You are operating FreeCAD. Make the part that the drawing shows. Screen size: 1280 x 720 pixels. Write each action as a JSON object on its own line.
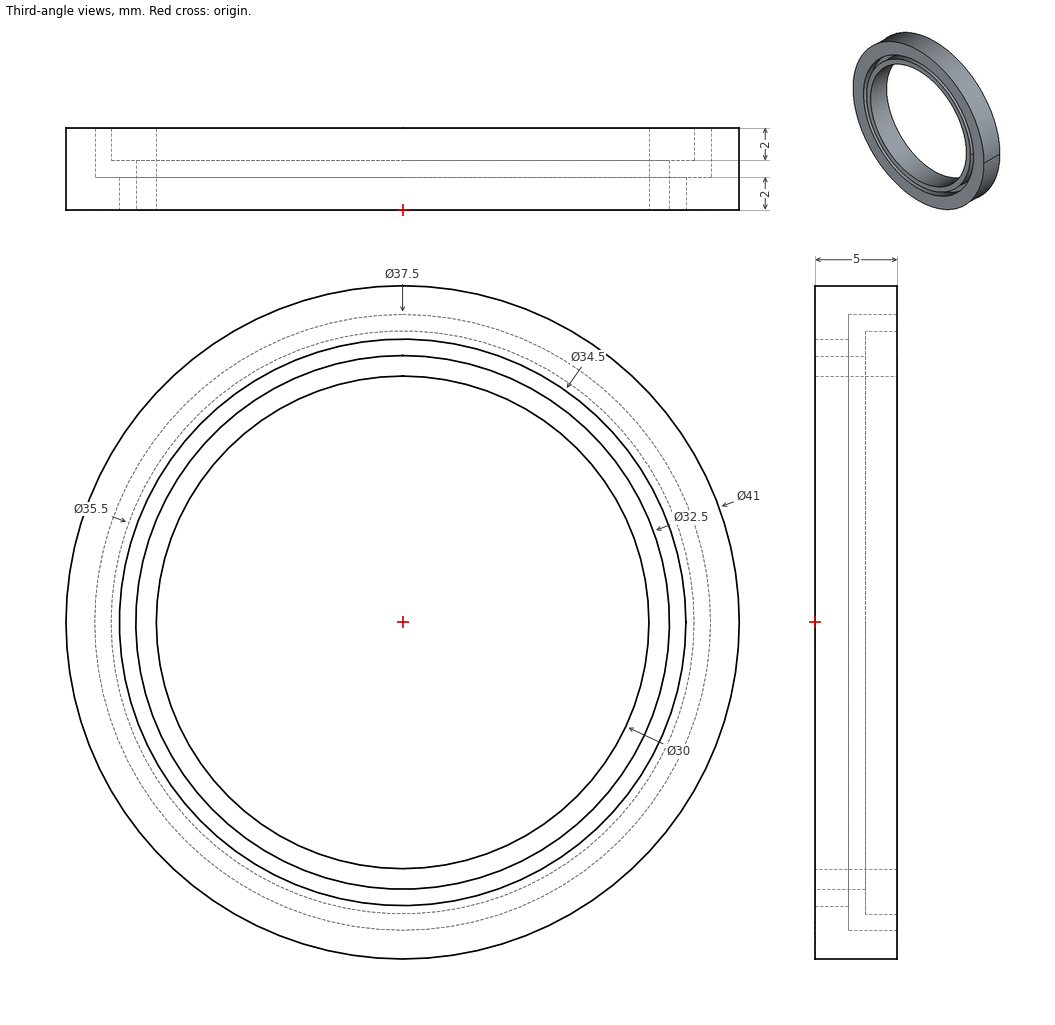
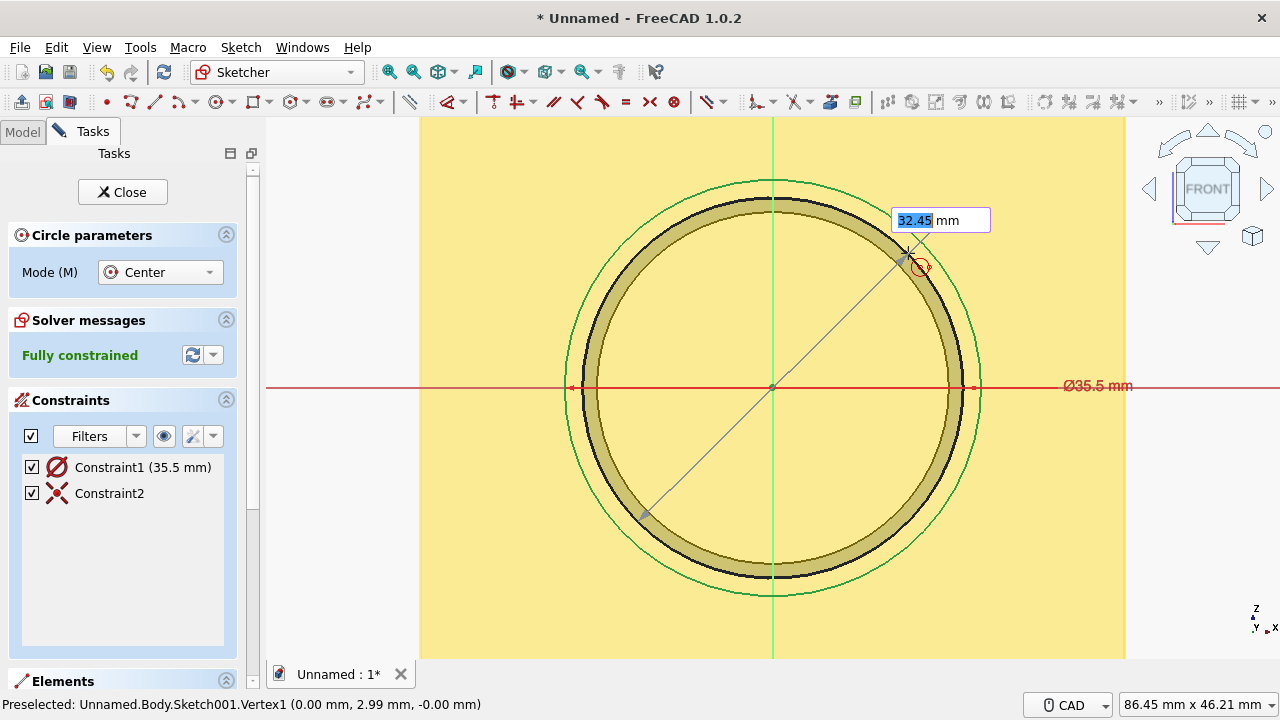
{"action": "type", "text": "32.5"}
{"action": "key", "text": "Return"}
{"action": "key", "text": "Escape"}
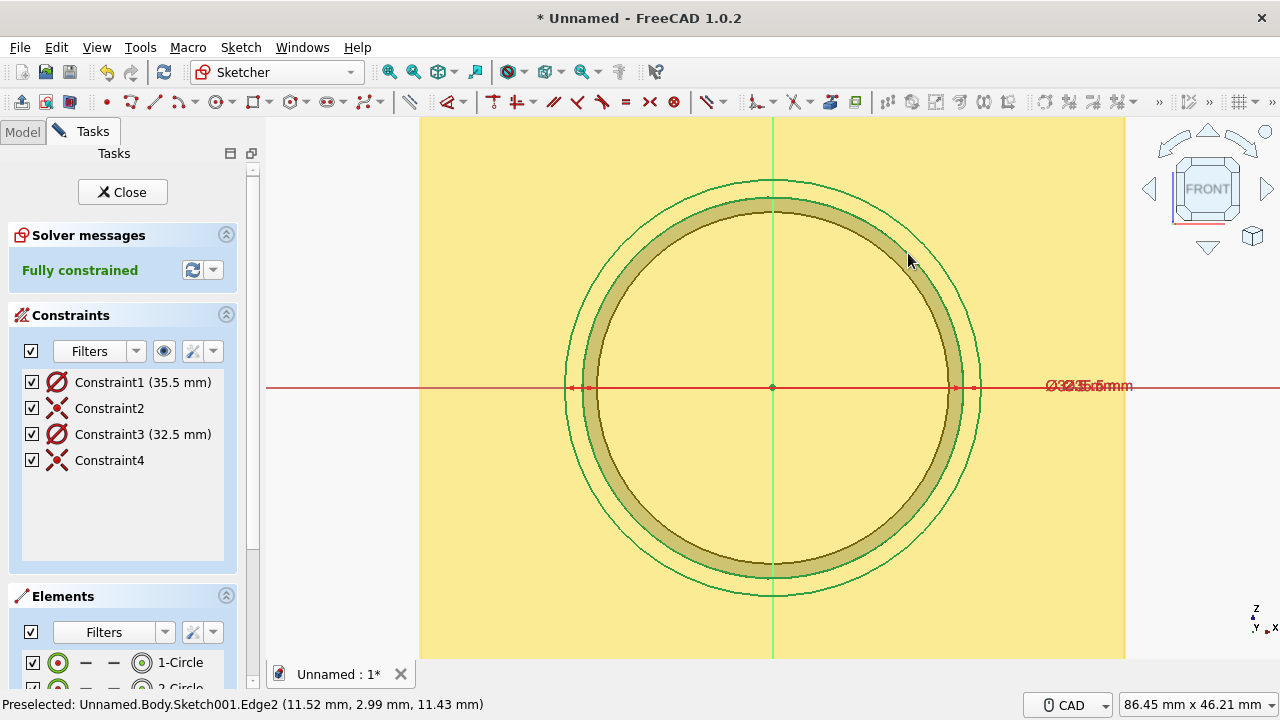
{"action": "left_click", "coordinate": [123, 192]}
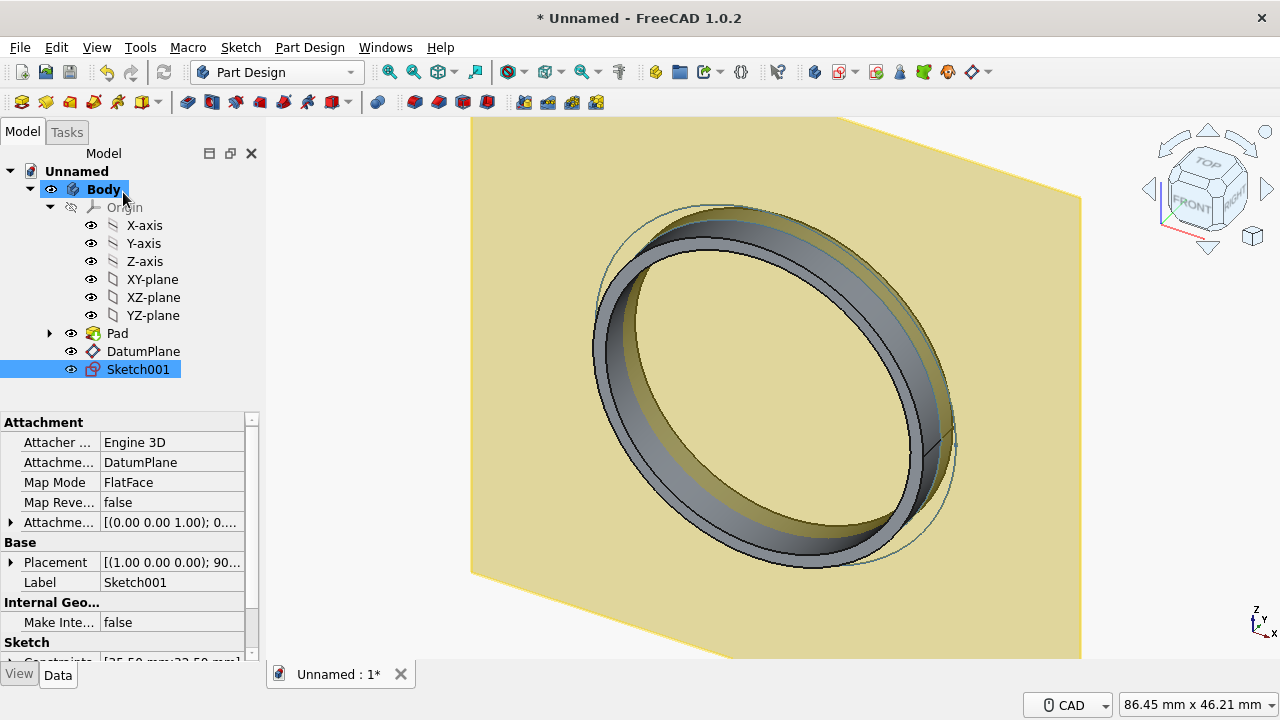
{"action": "left_click", "coordinate": [22, 102]}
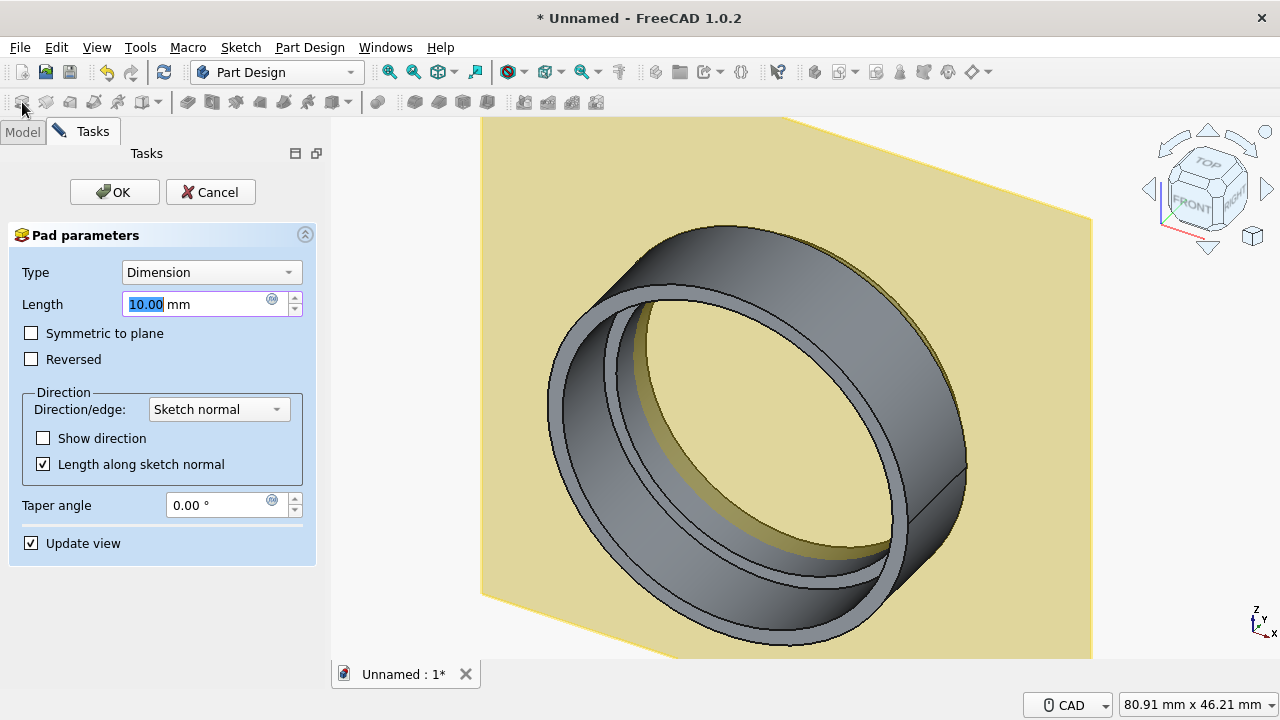
{"action": "type", "text": "2"}
{"action": "key", "text": "Tab"}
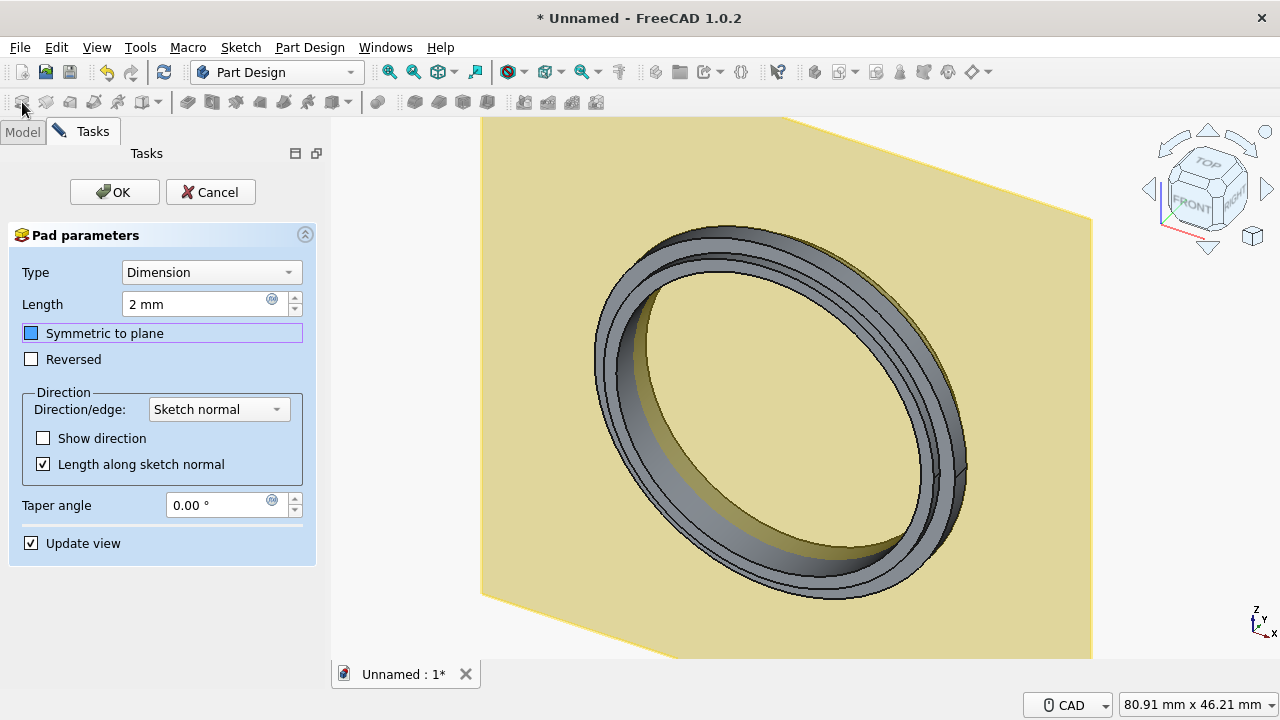
{"action": "left_click", "coordinate": [30, 359]}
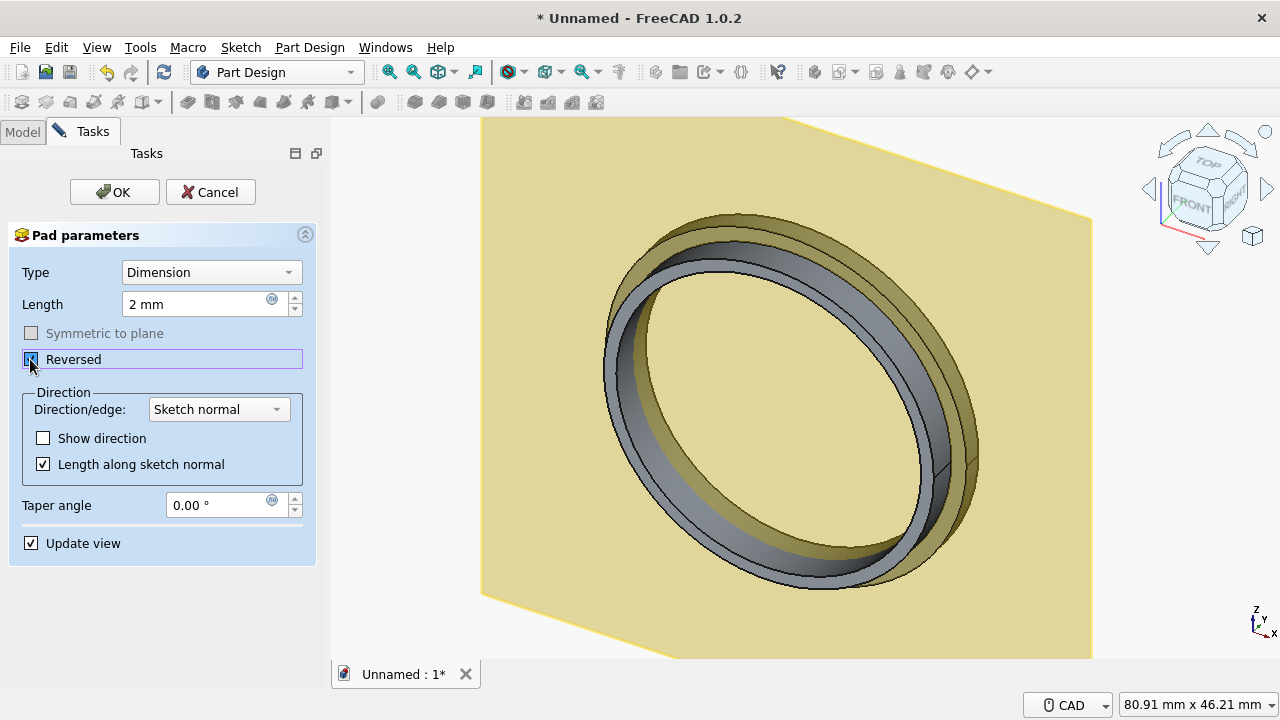
{"action": "left_click", "coordinate": [115, 192]}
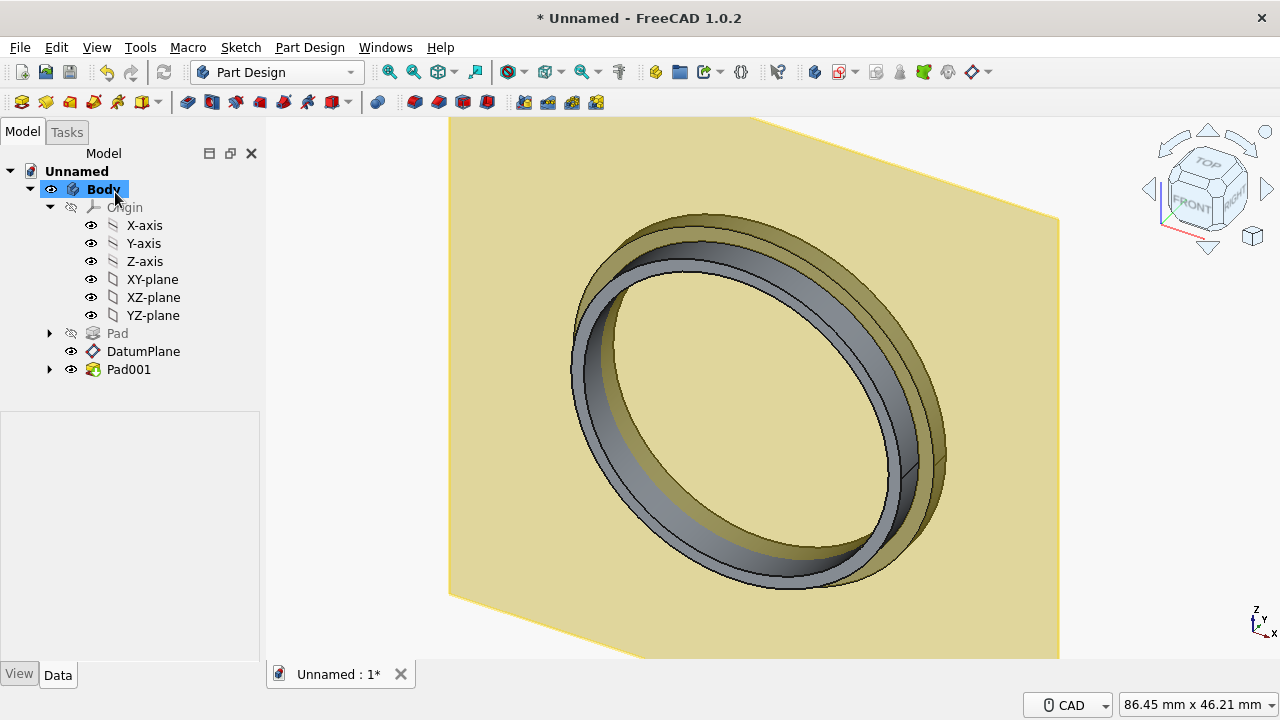
{"action": "left_click", "coordinate": [116, 351]}
{"action": "key", "text": "space"}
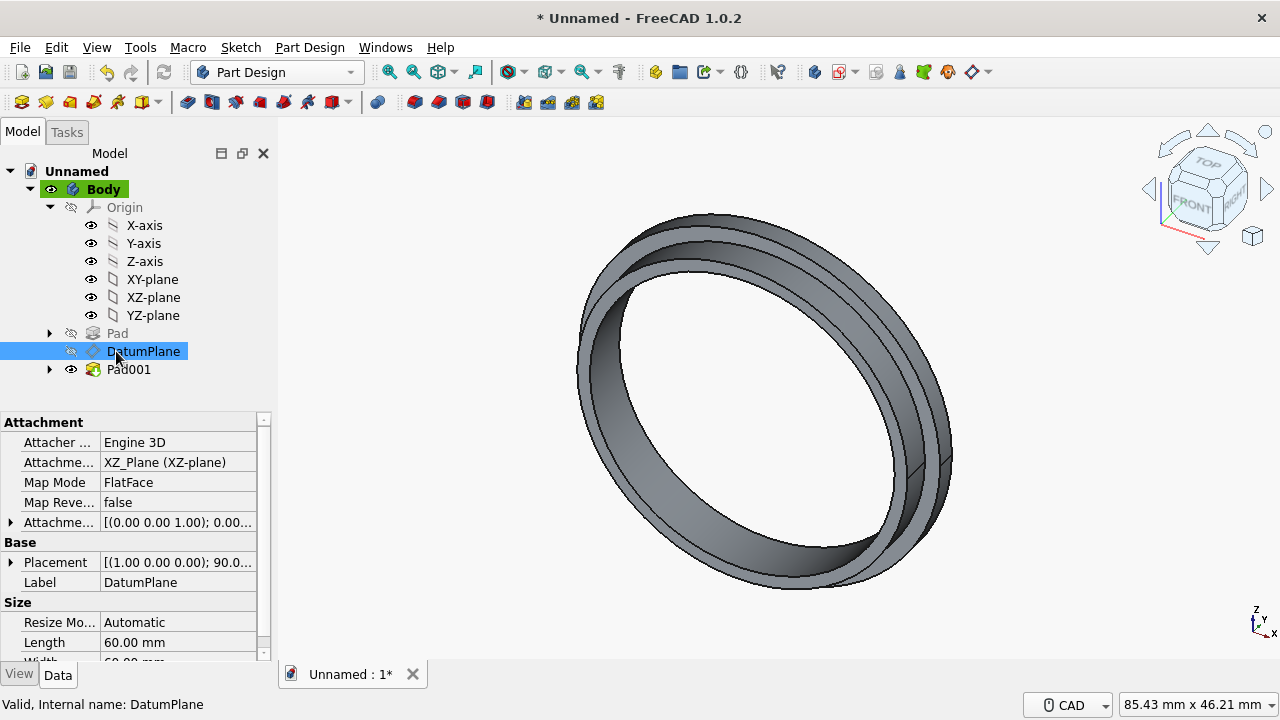
{"action": "left_click", "coordinate": [318, 619]}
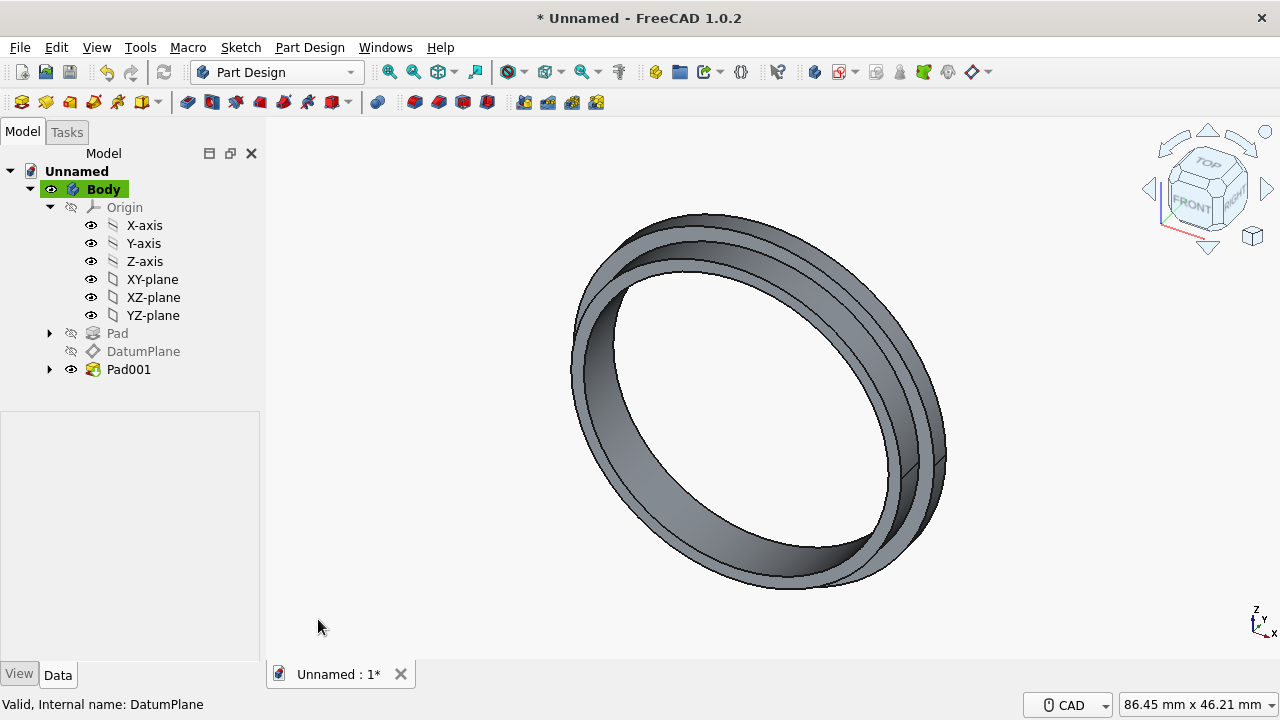
{"action": "left_click", "coordinate": [816, 72]}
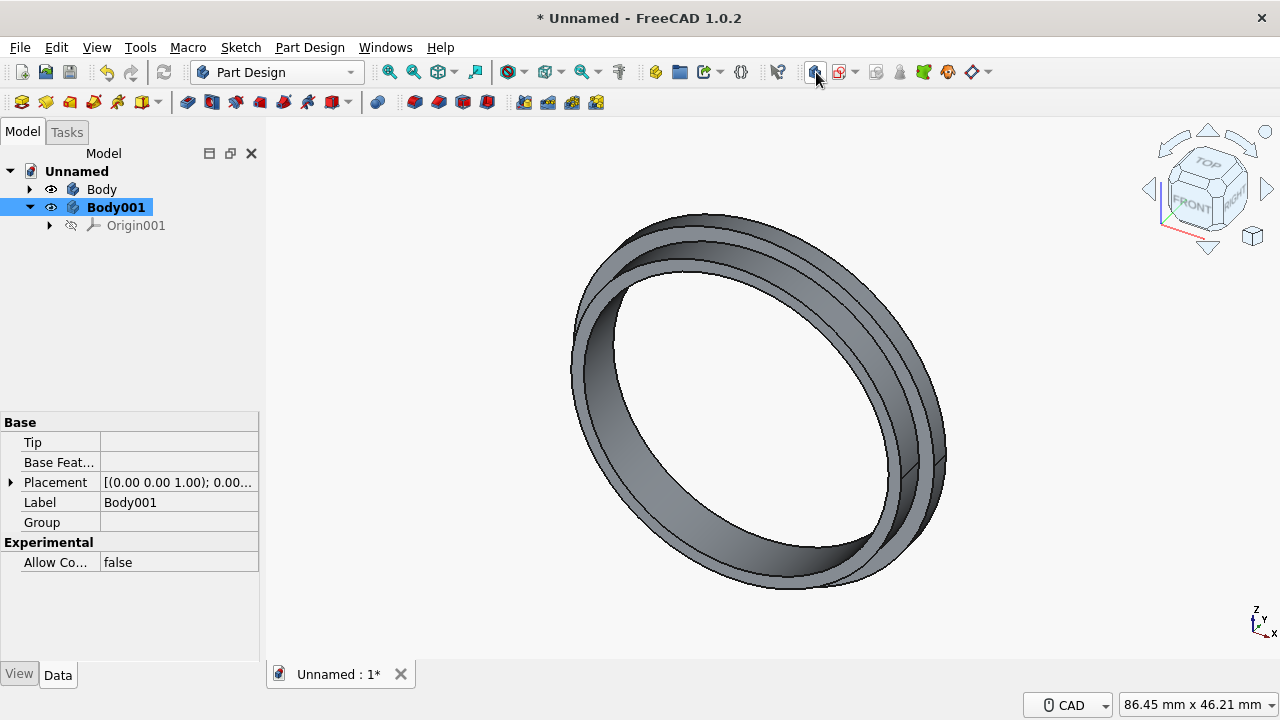
{"action": "left_click", "coordinate": [306, 619]}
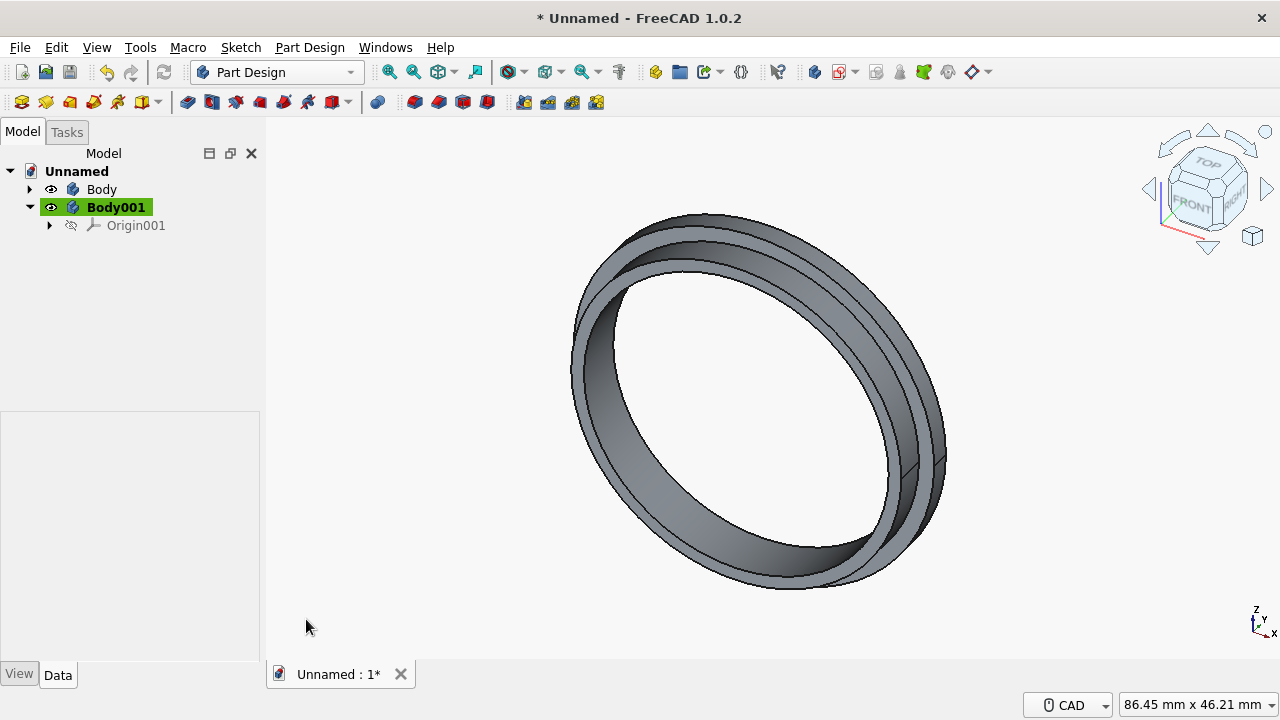
{"action": "left_click", "coordinate": [840, 72]}